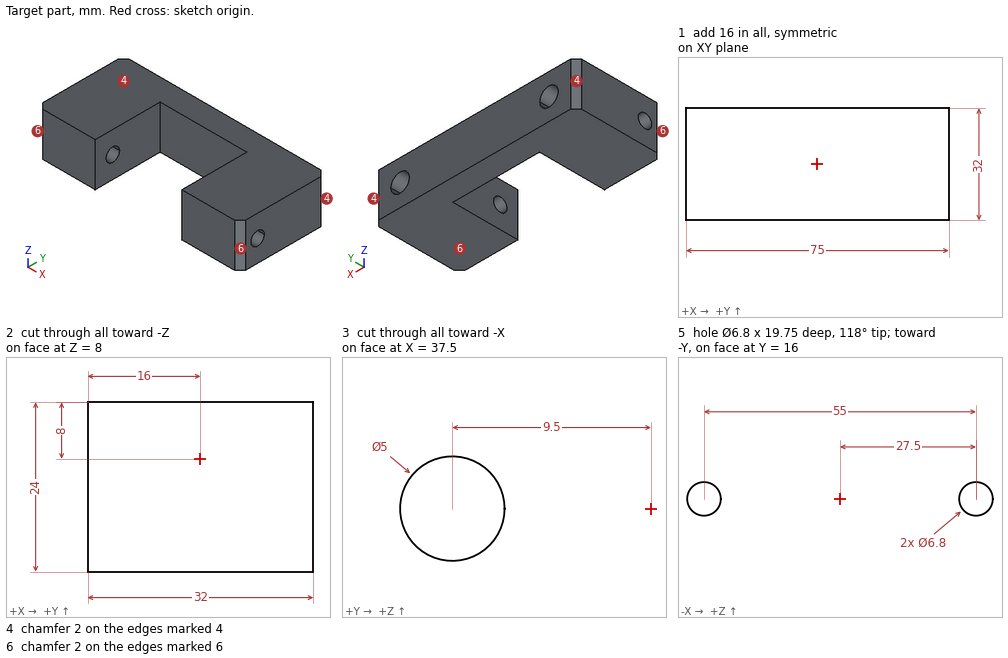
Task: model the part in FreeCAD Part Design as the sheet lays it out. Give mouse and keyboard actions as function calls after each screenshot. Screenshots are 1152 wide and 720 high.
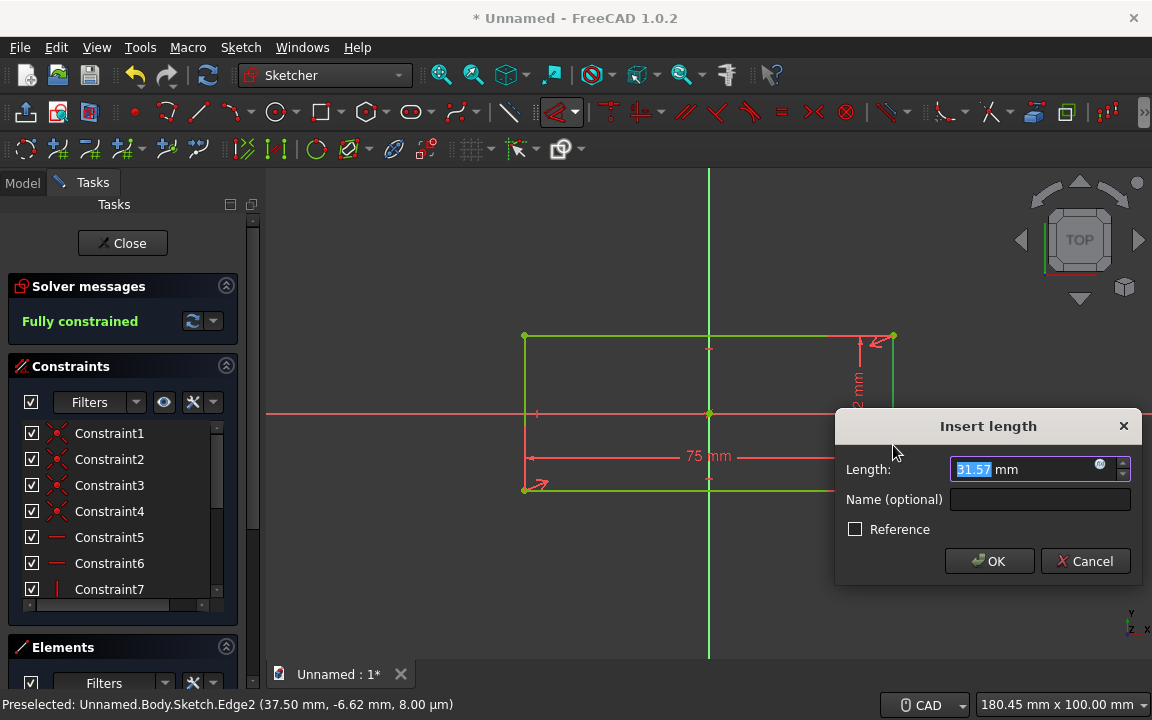
text(32)
key(Return)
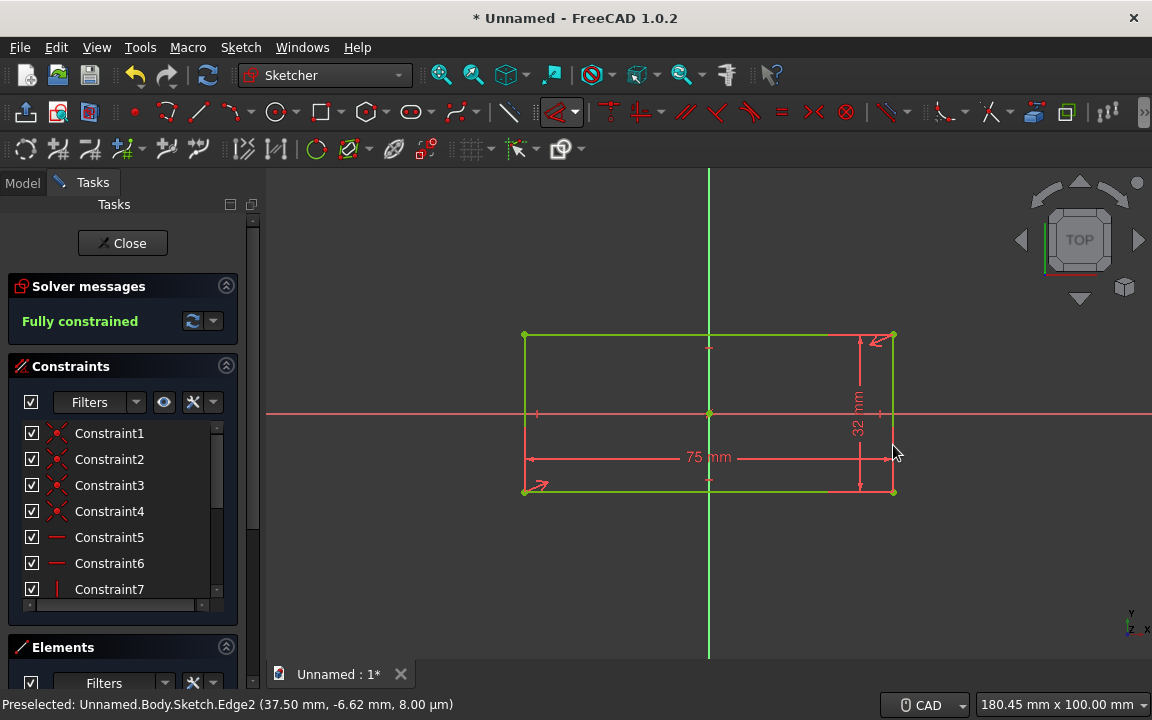
click(123, 243)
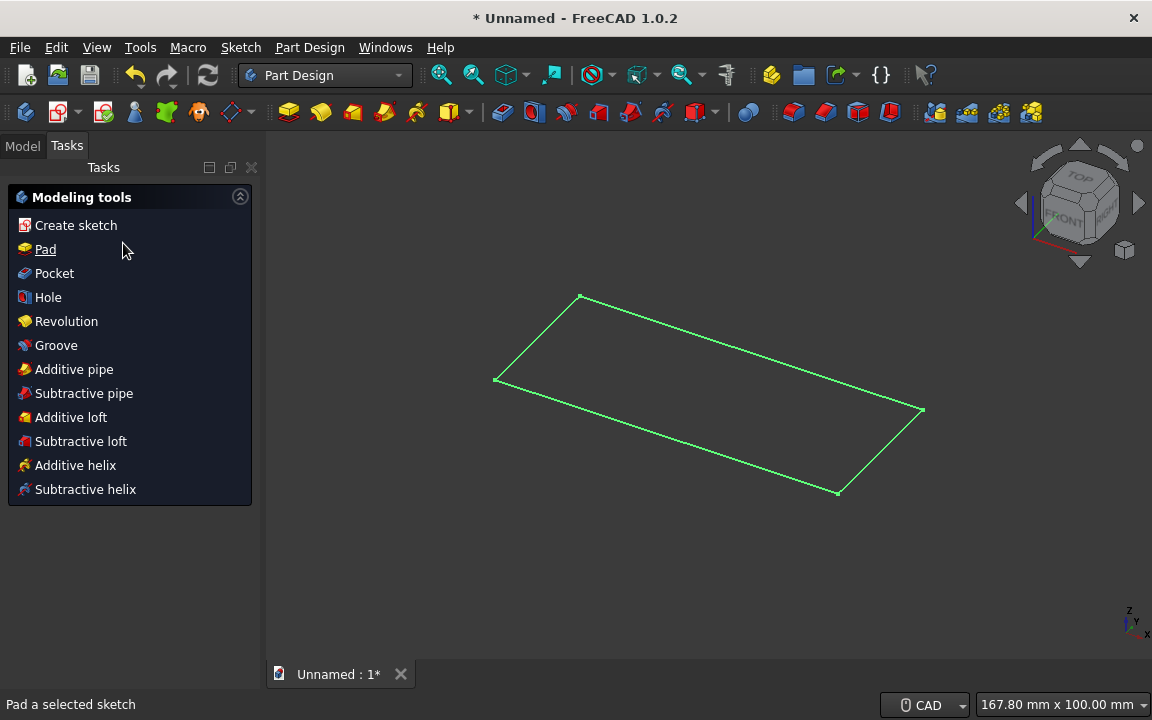
click(290, 112)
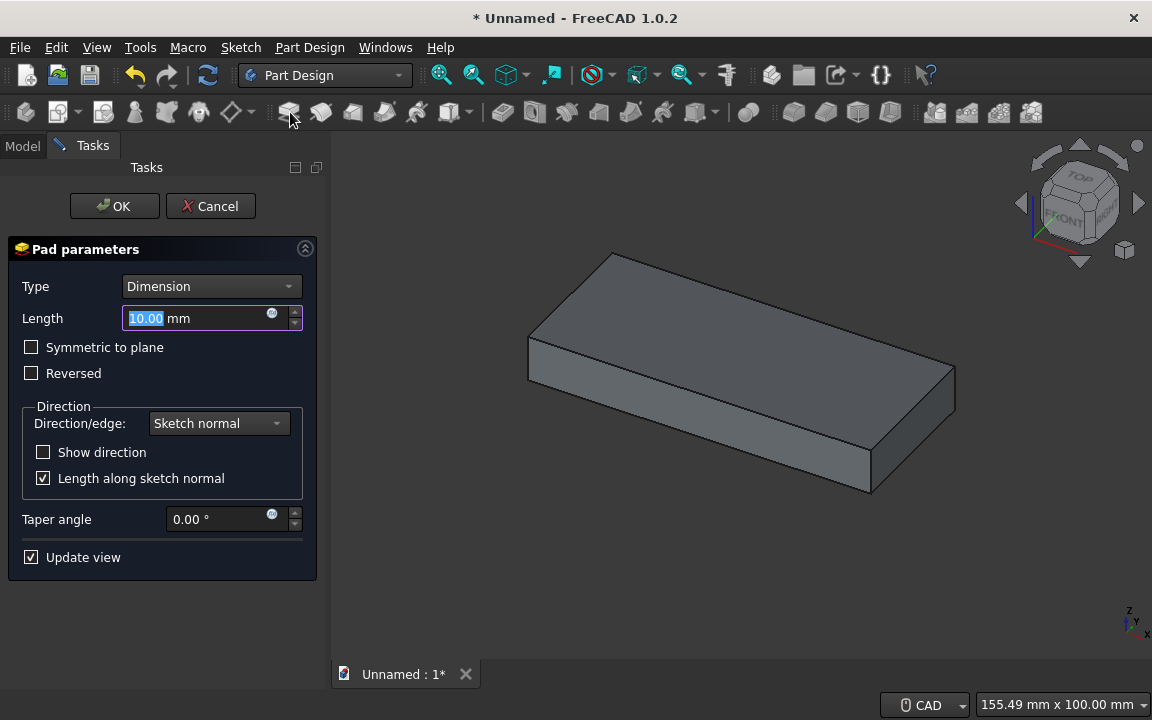
text(16)
key(Tab)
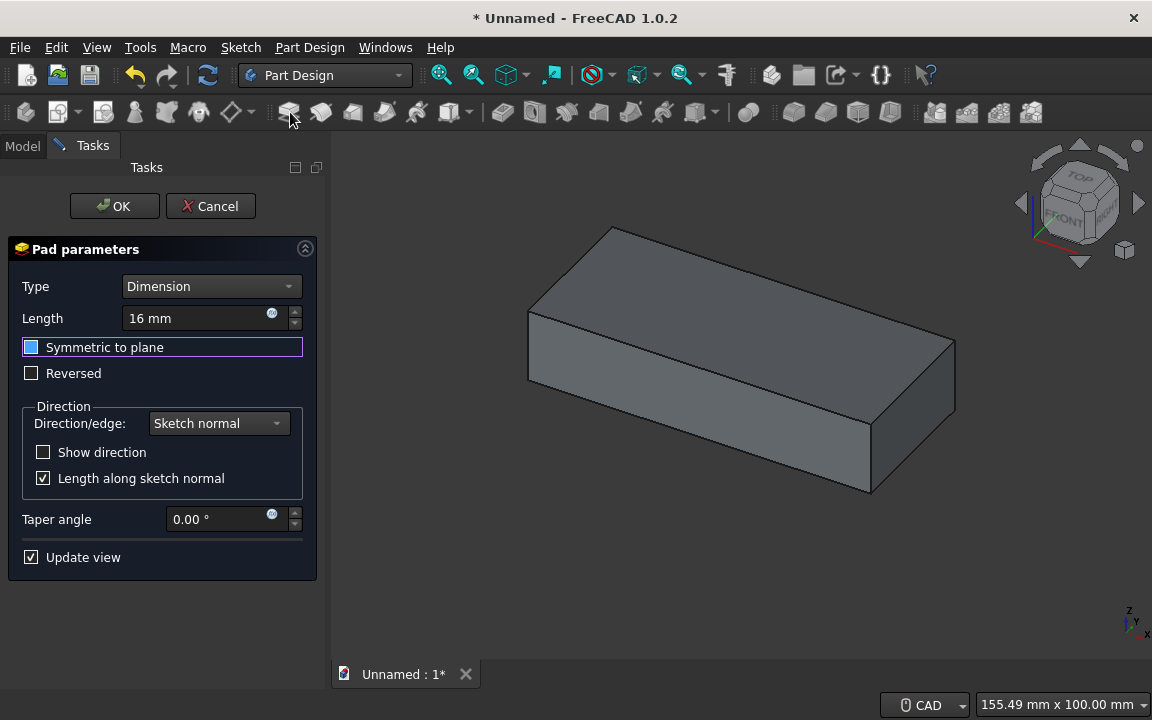
click(30, 347)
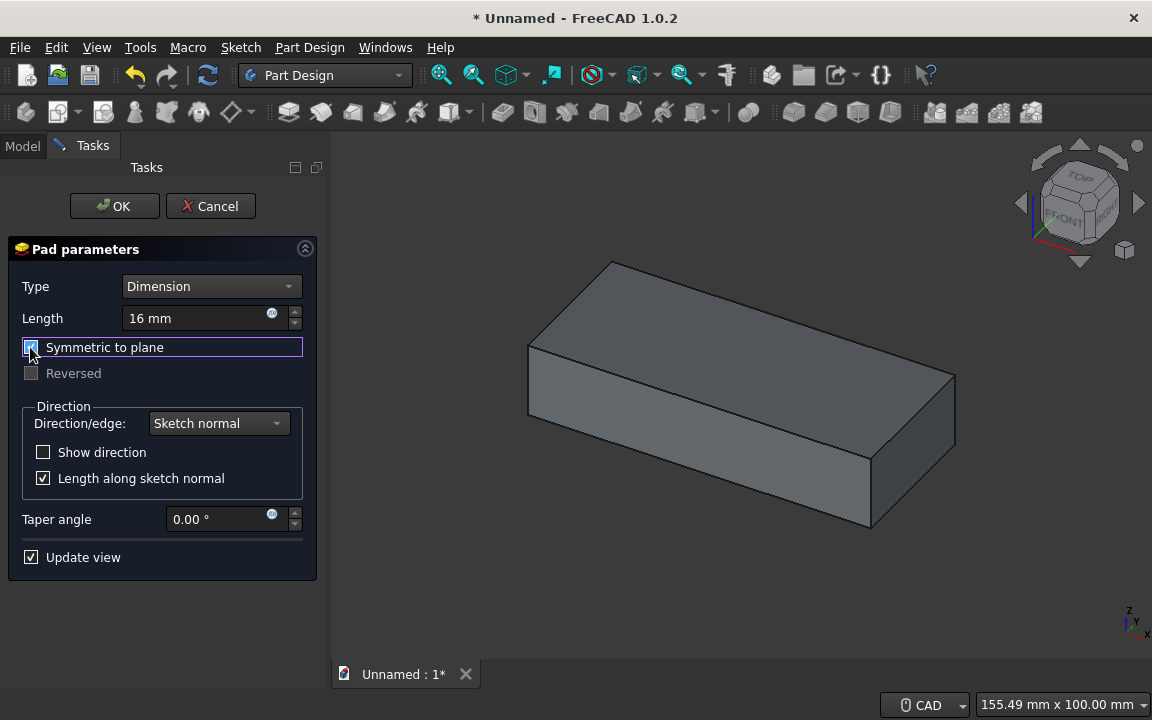
click(115, 206)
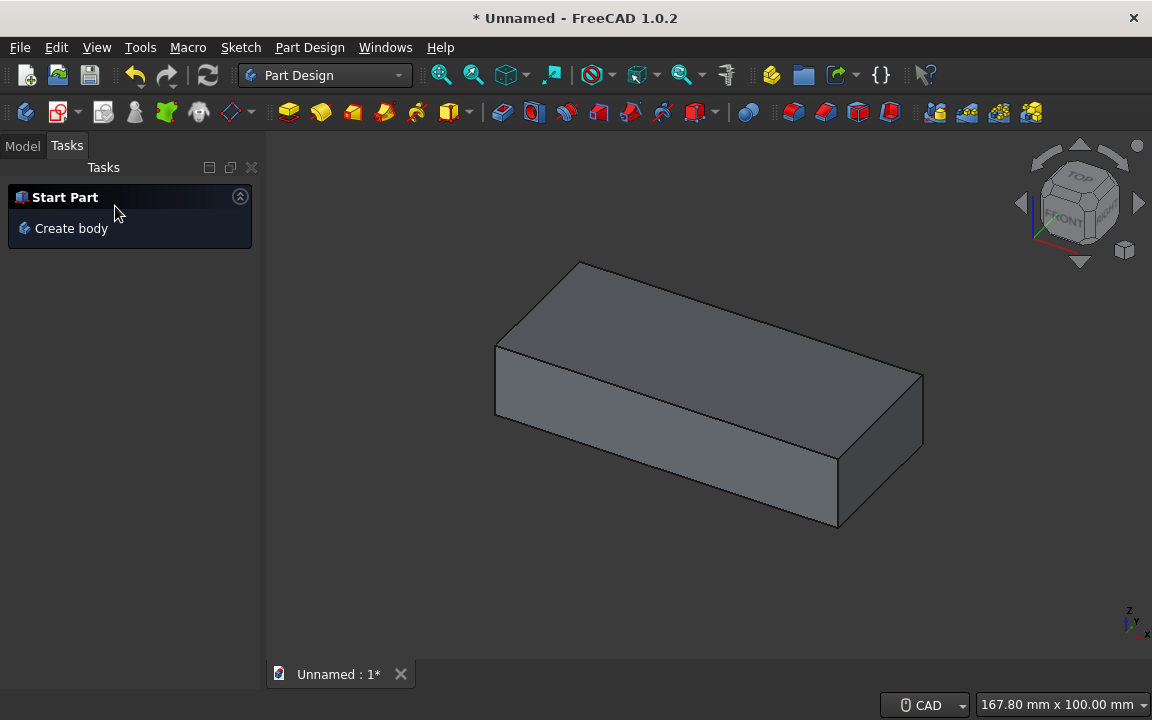
click(807, 392)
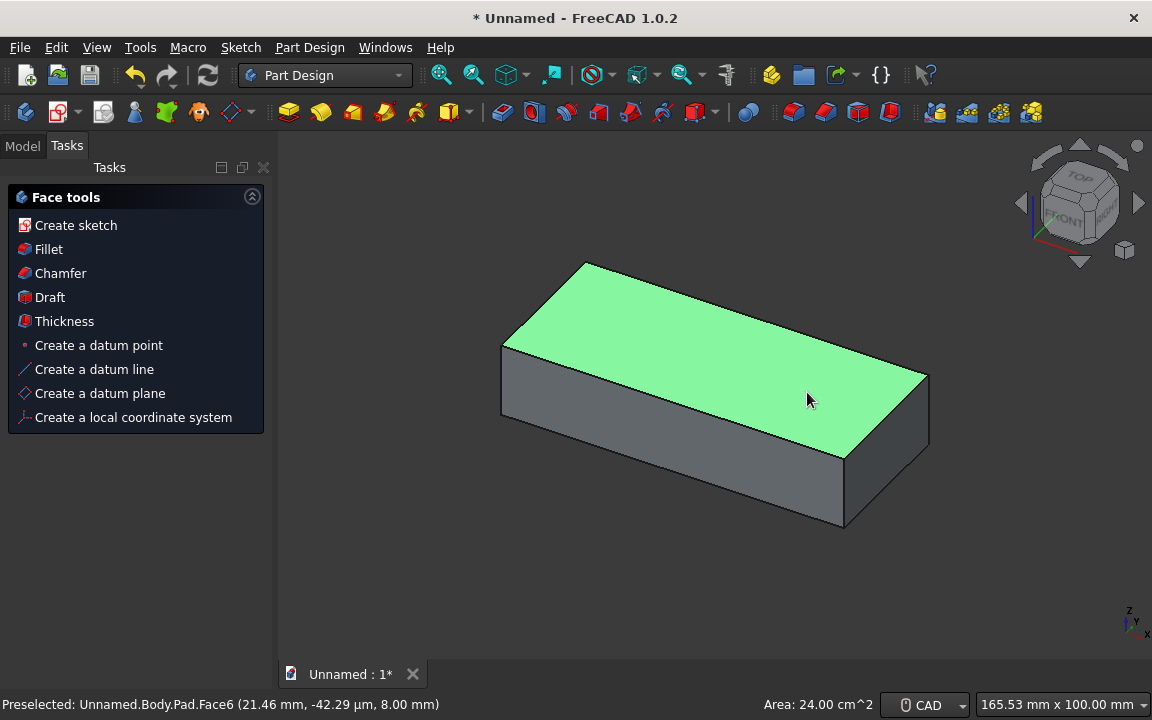
click(58, 112)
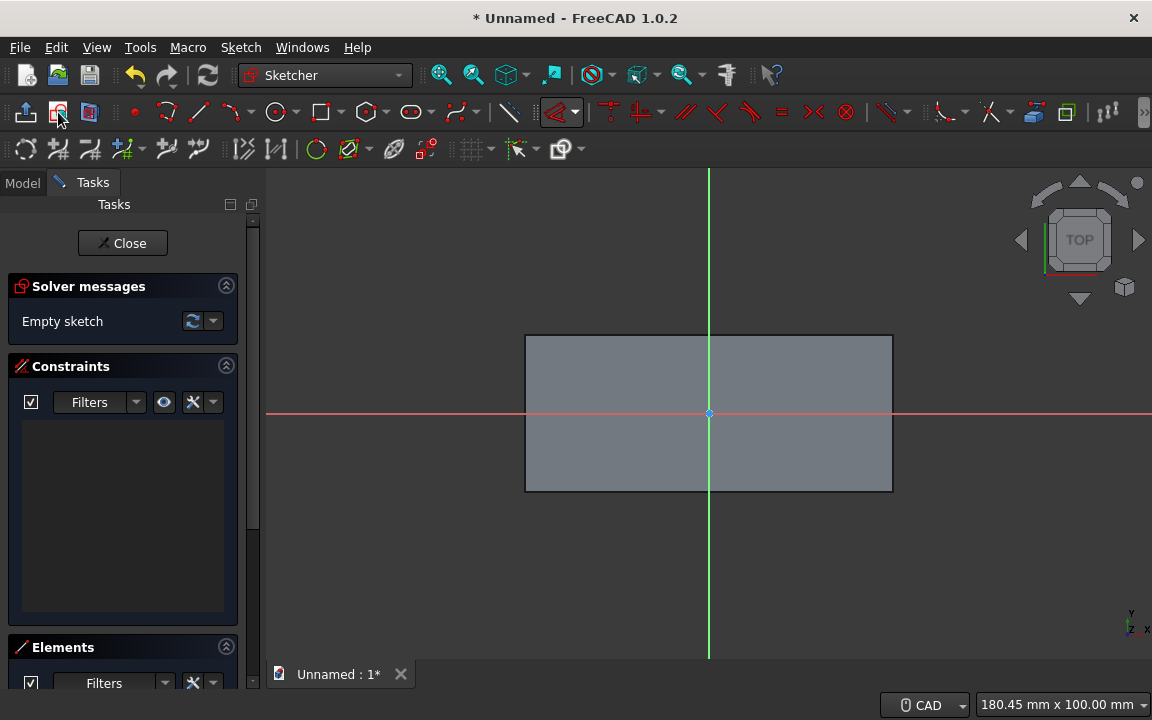
scroll(749, 445, up, 5)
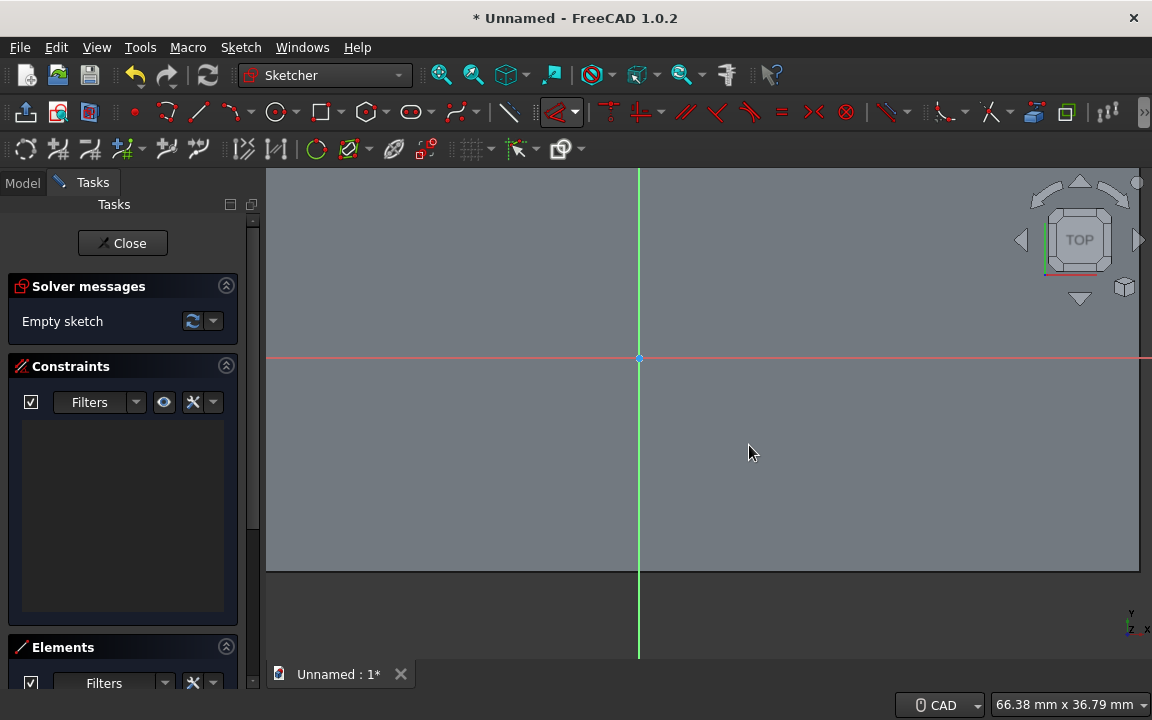
key(g)
key(r)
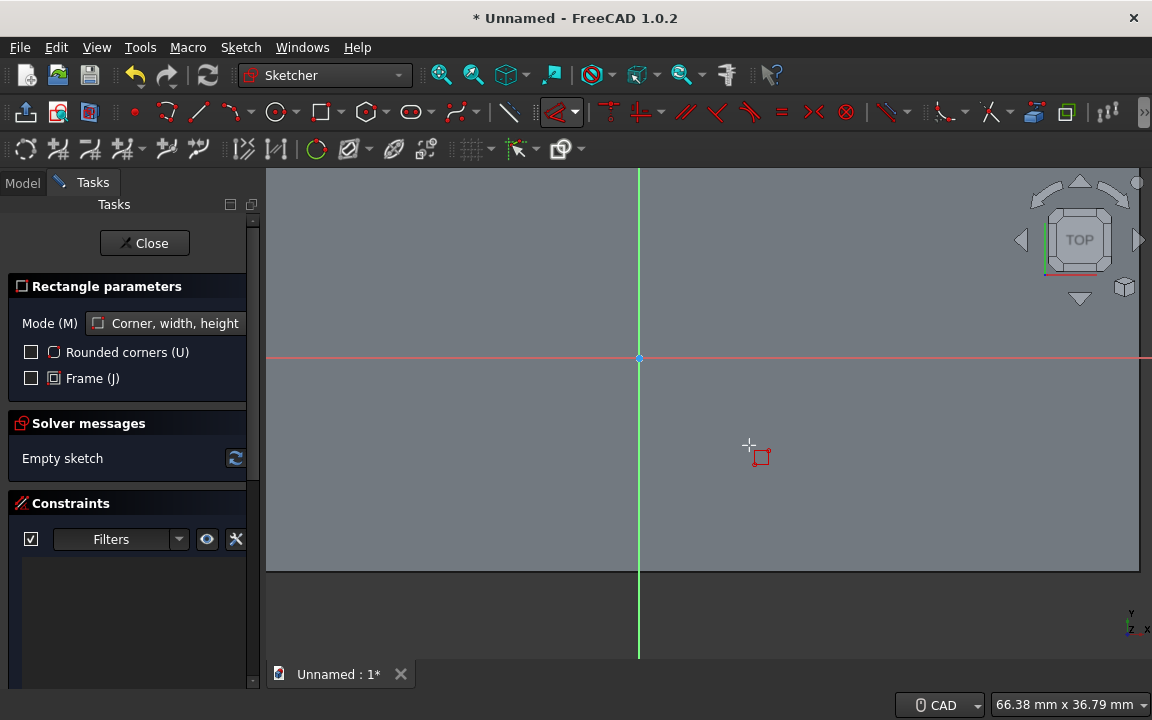
click(426, 252)
click(853, 572)
key(Escape)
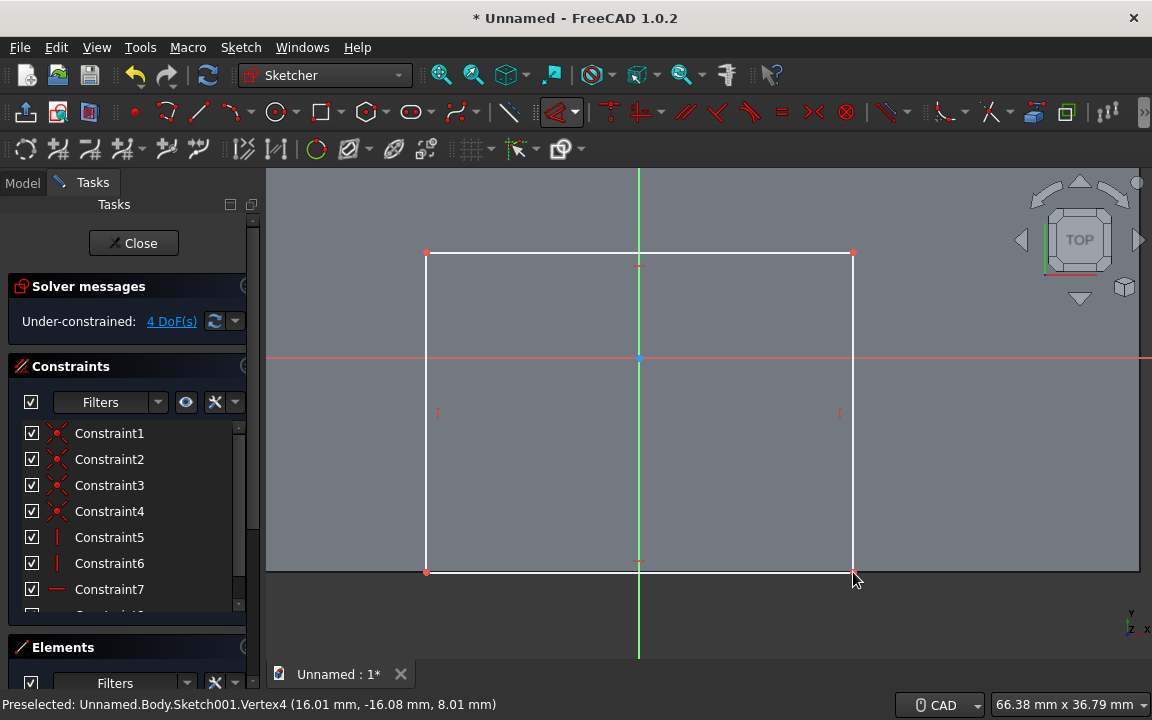
scroll(426, 349, up, 2)